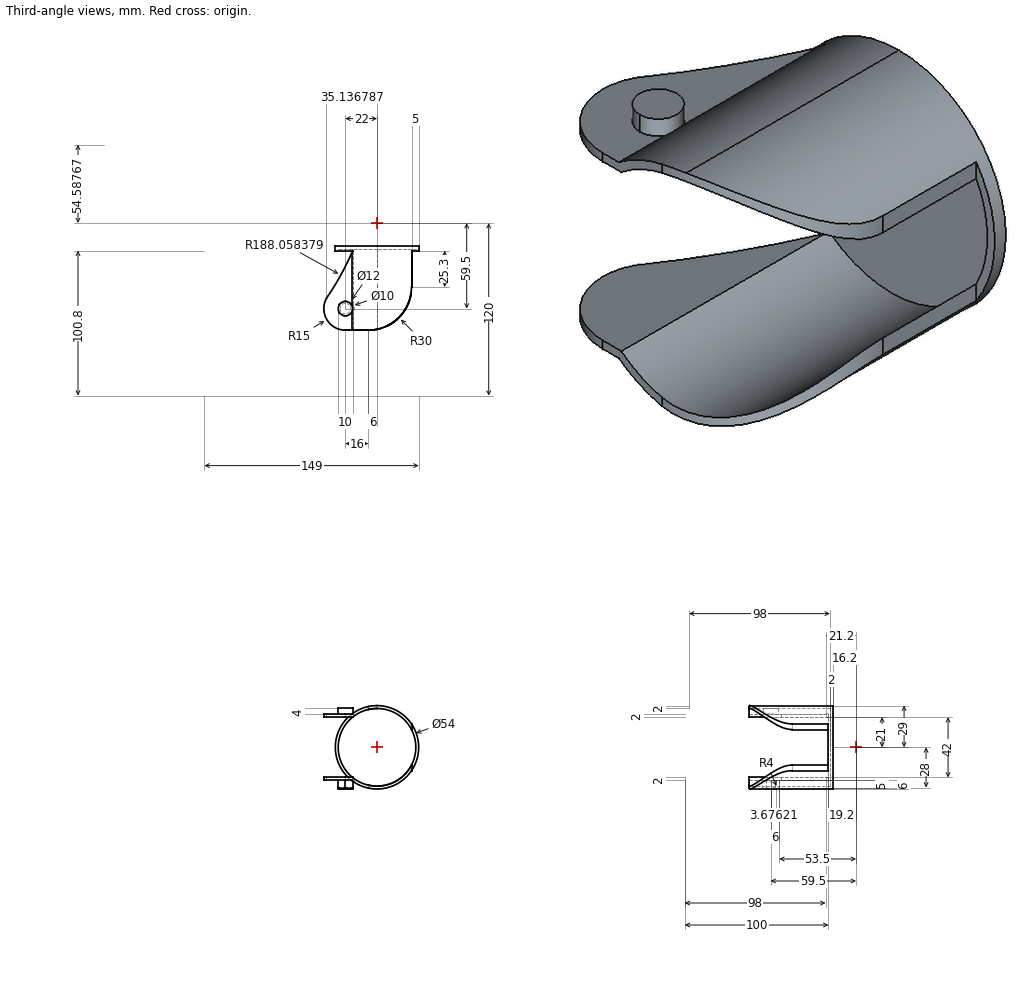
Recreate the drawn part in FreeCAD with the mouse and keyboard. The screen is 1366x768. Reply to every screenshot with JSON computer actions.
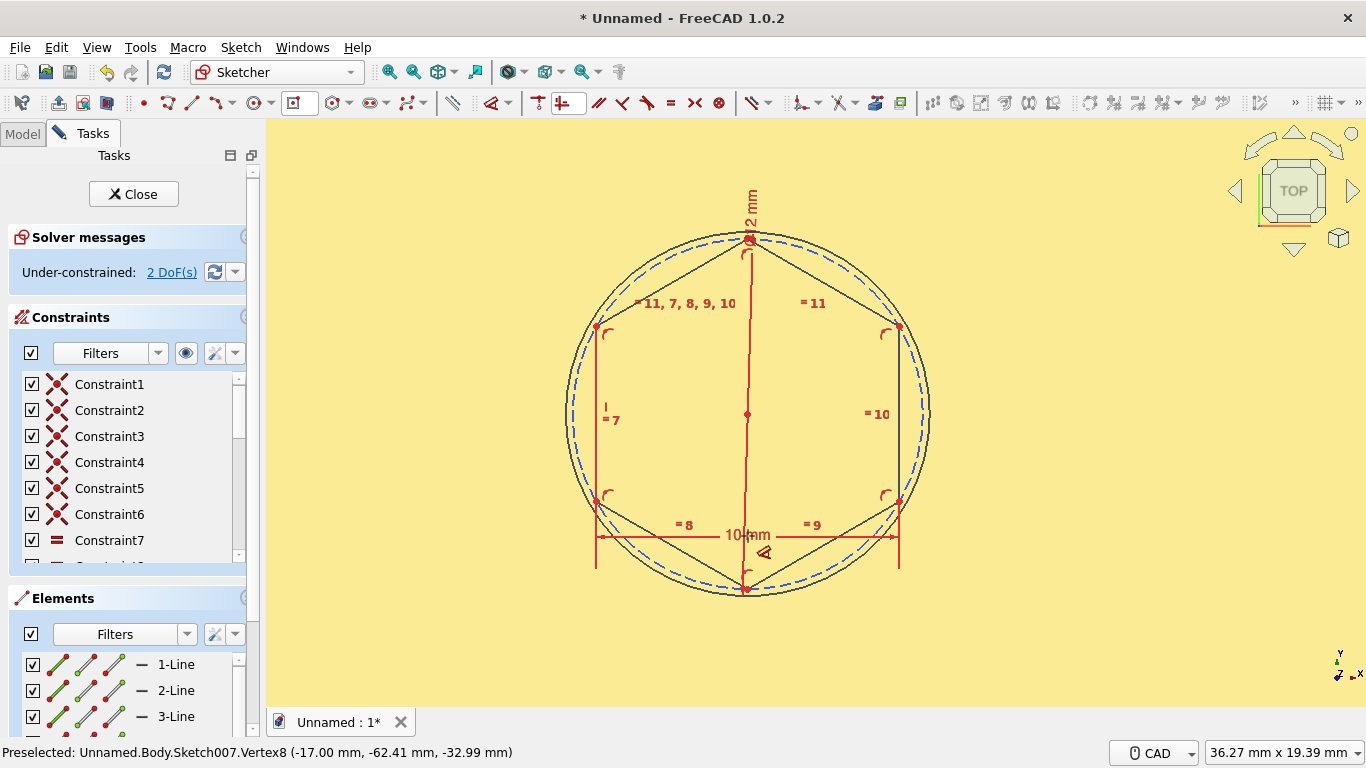
{"action": "left_click", "coordinate": [748, 414]}
{"action": "left_click", "coordinate": [974, 448]}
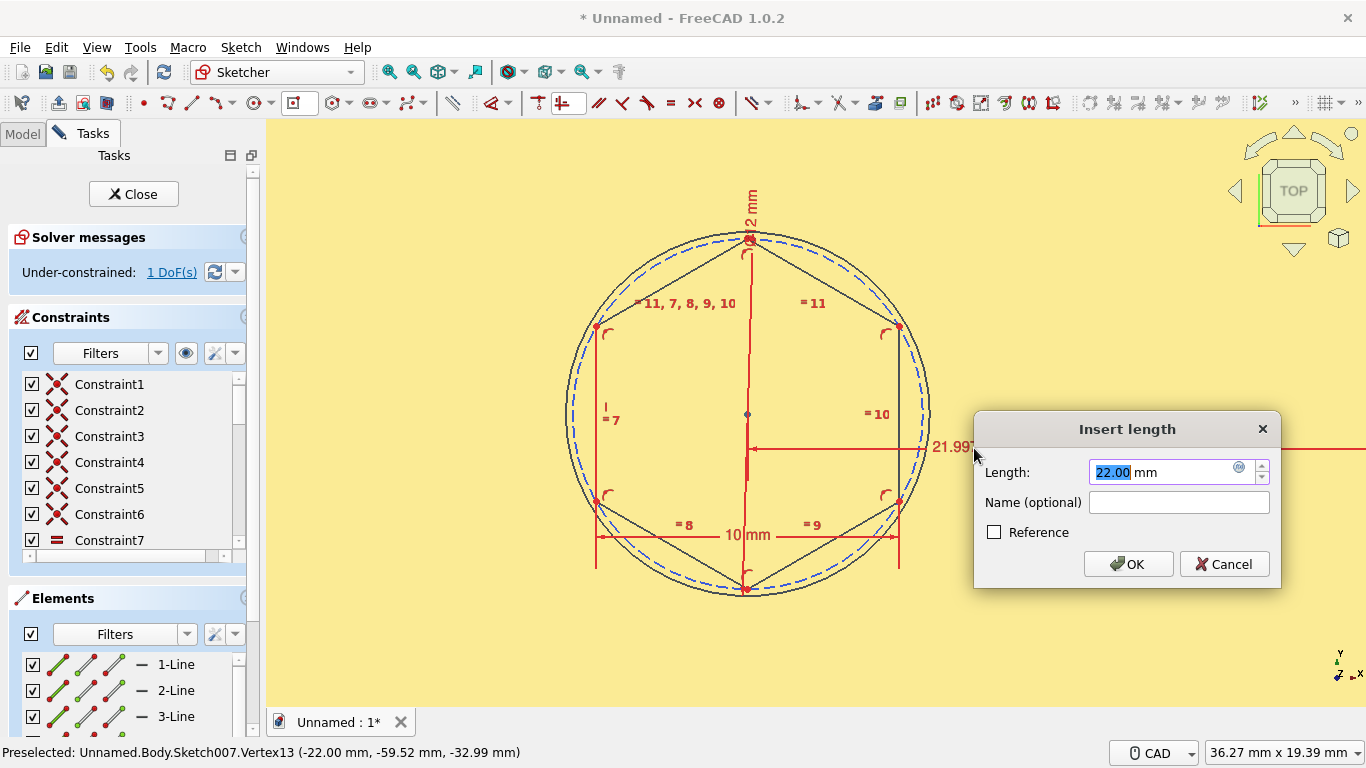
{"action": "type", "text": "22"}
{"action": "key", "text": "Return"}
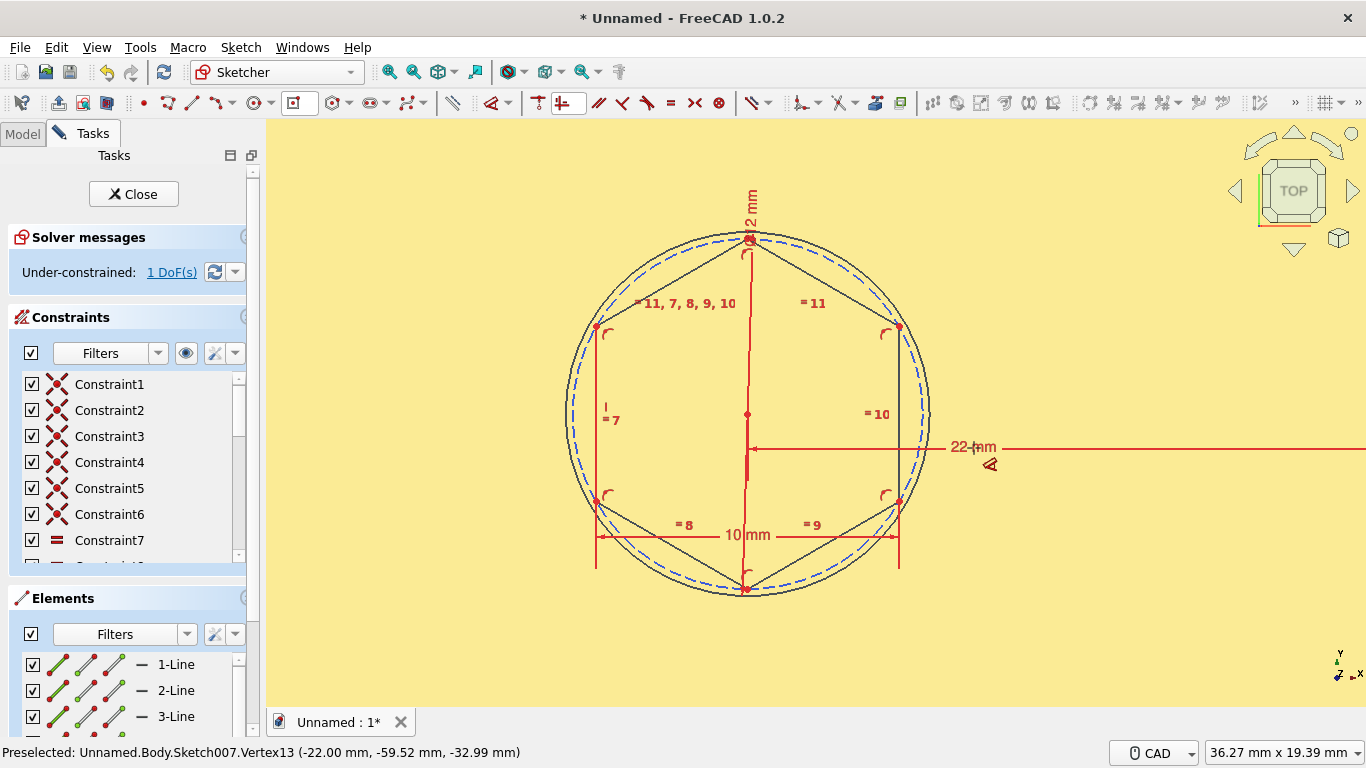
{"action": "left_click", "coordinate": [748, 414]}
{"action": "left_click", "coordinate": [714, 281]}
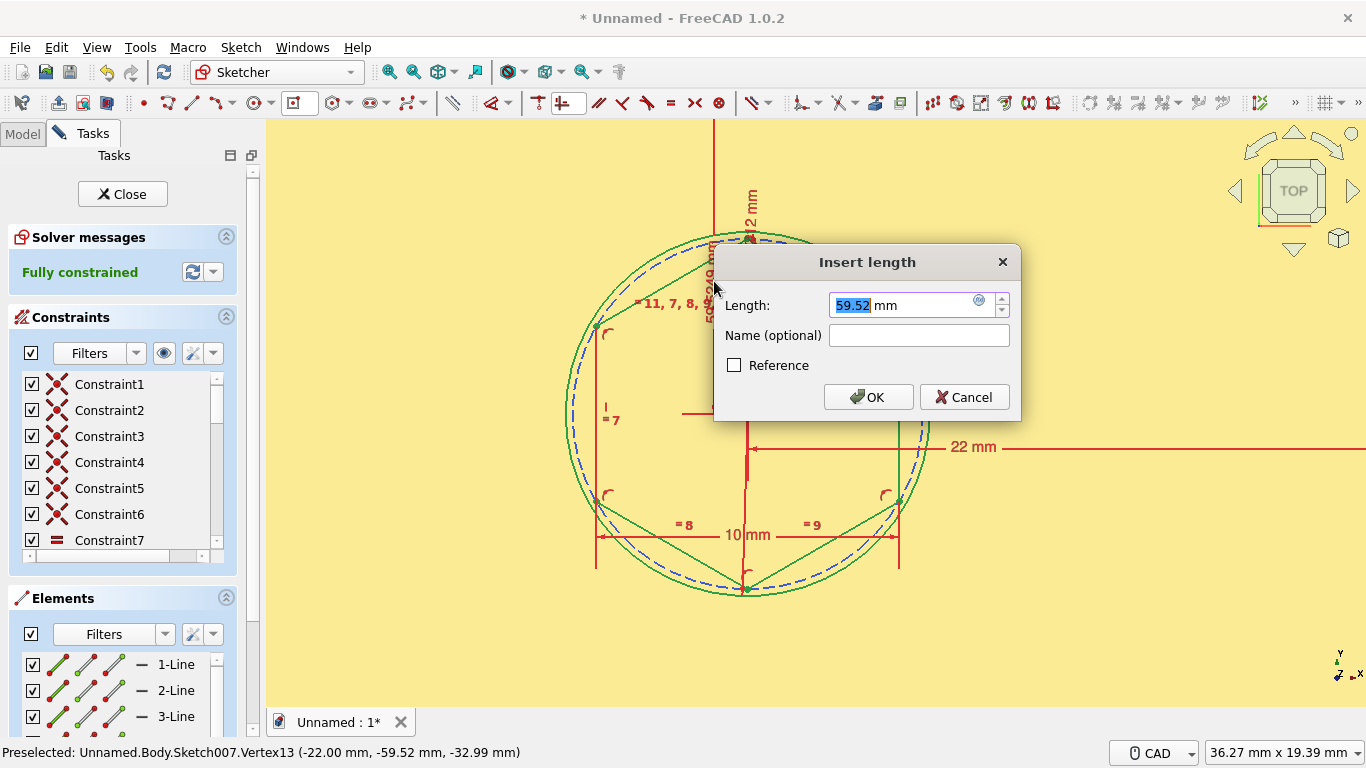
{"action": "type", "text": "59.5"}
{"action": "key", "text": "Return"}
{"action": "key", "text": "Escape"}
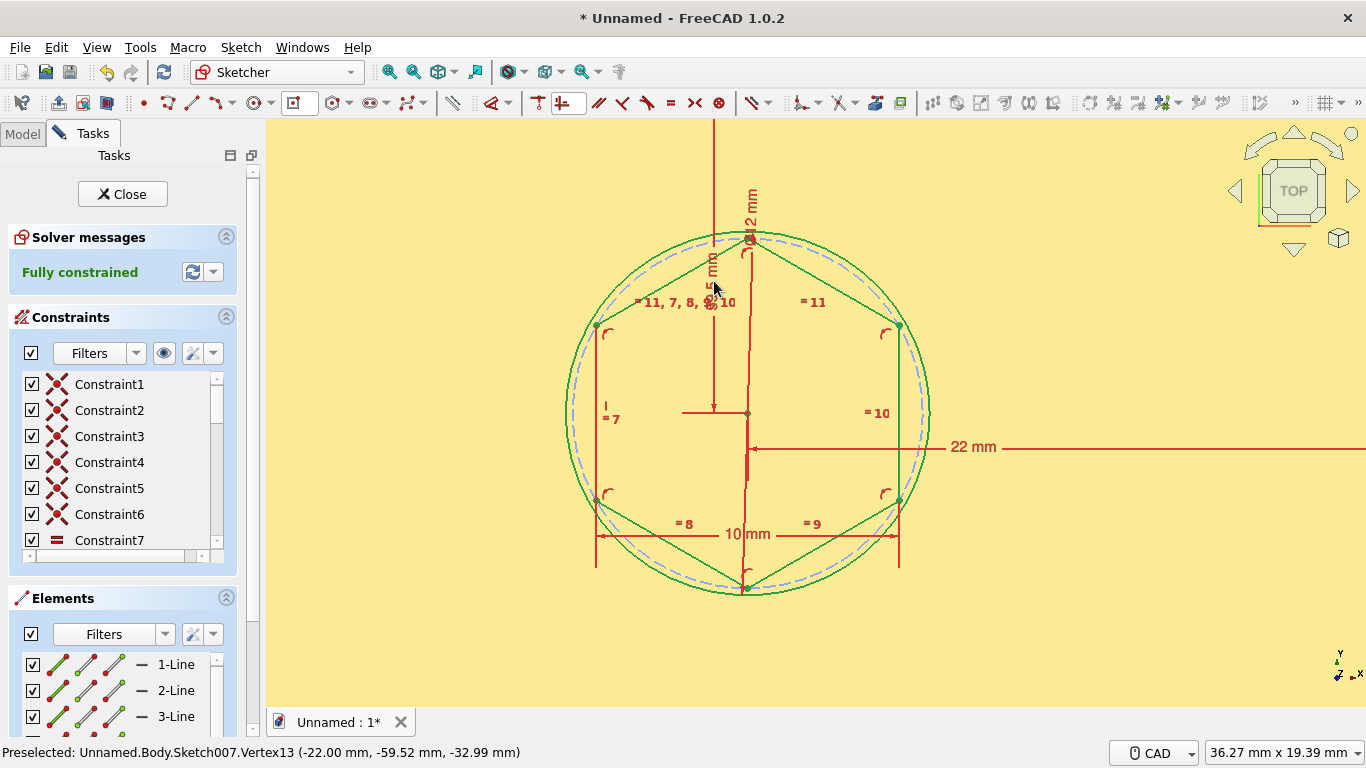
{"action": "left_click", "coordinate": [123, 194]}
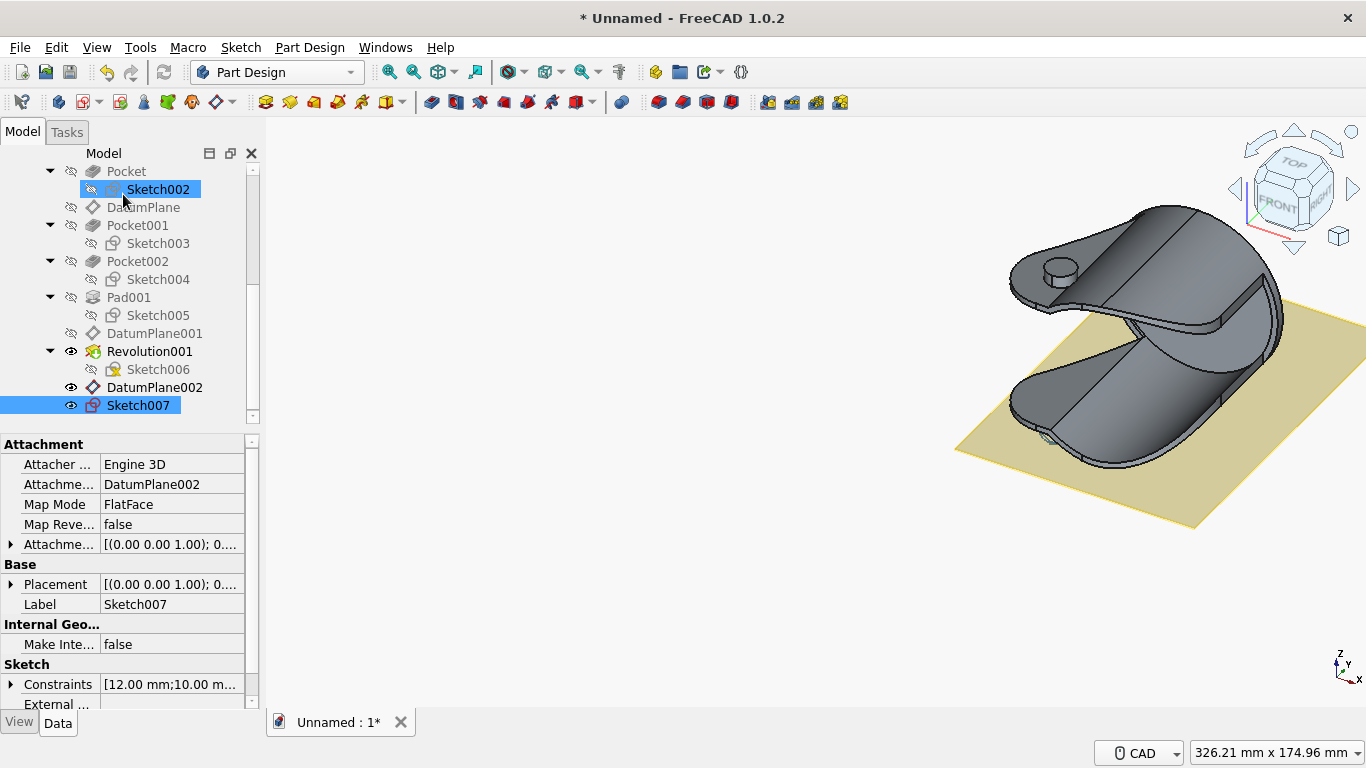
{"action": "left_click", "coordinate": [432, 102]}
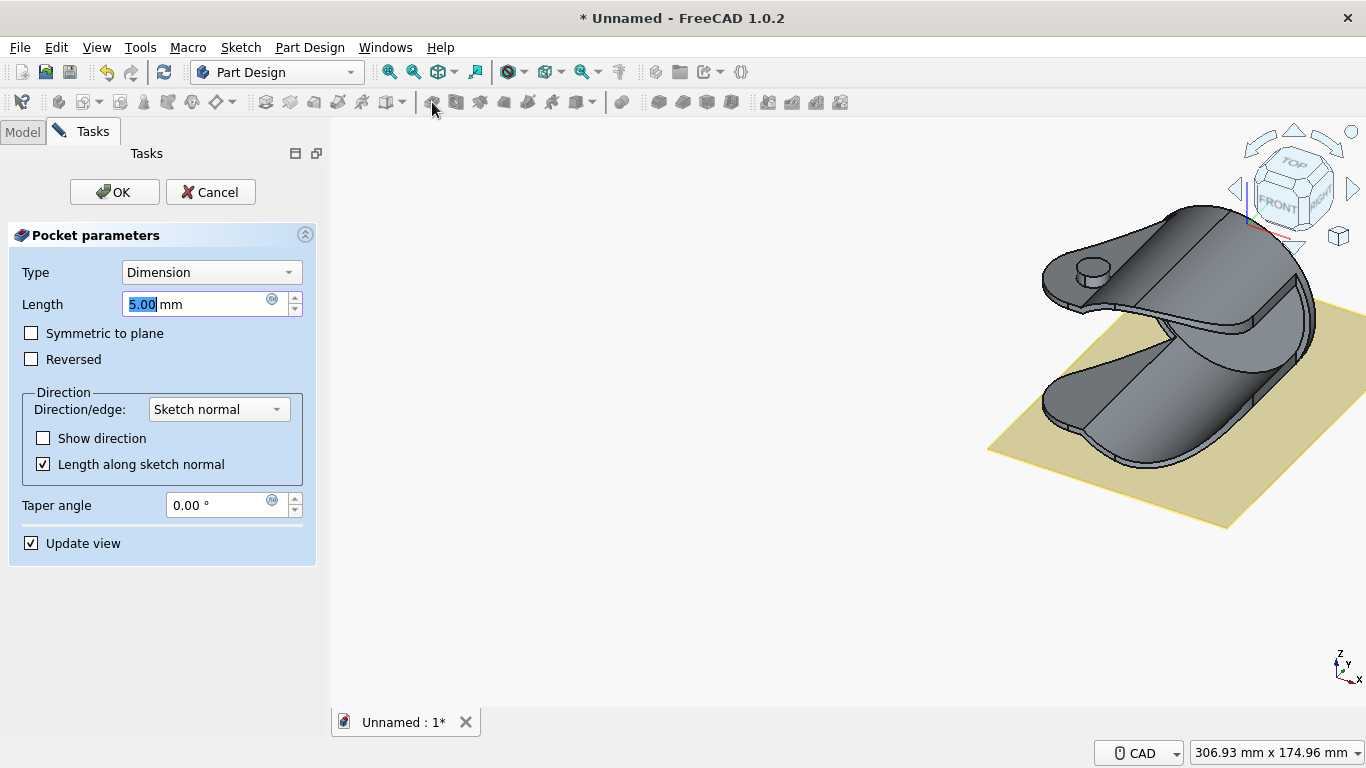
{"action": "type", "text": "10"}
{"action": "key", "text": "Tab"}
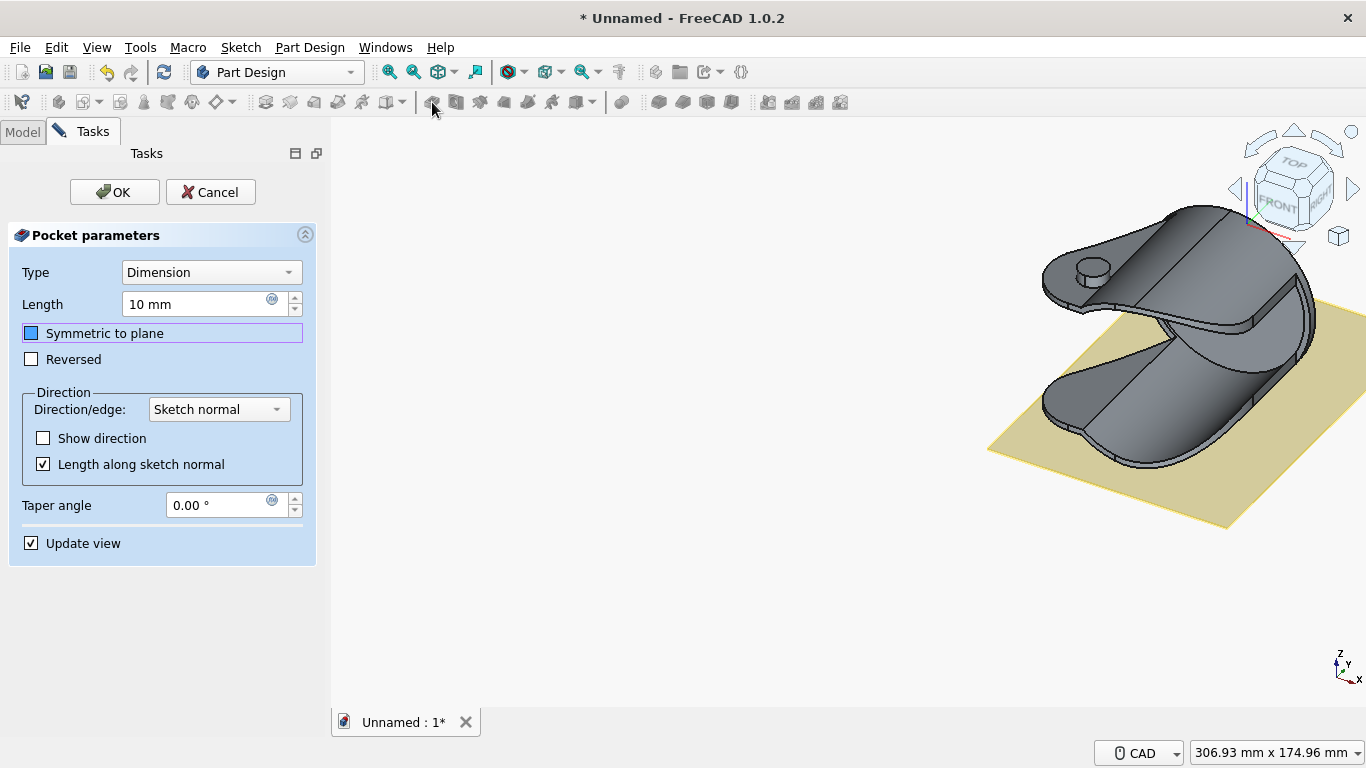
{"action": "left_click", "coordinate": [30, 359]}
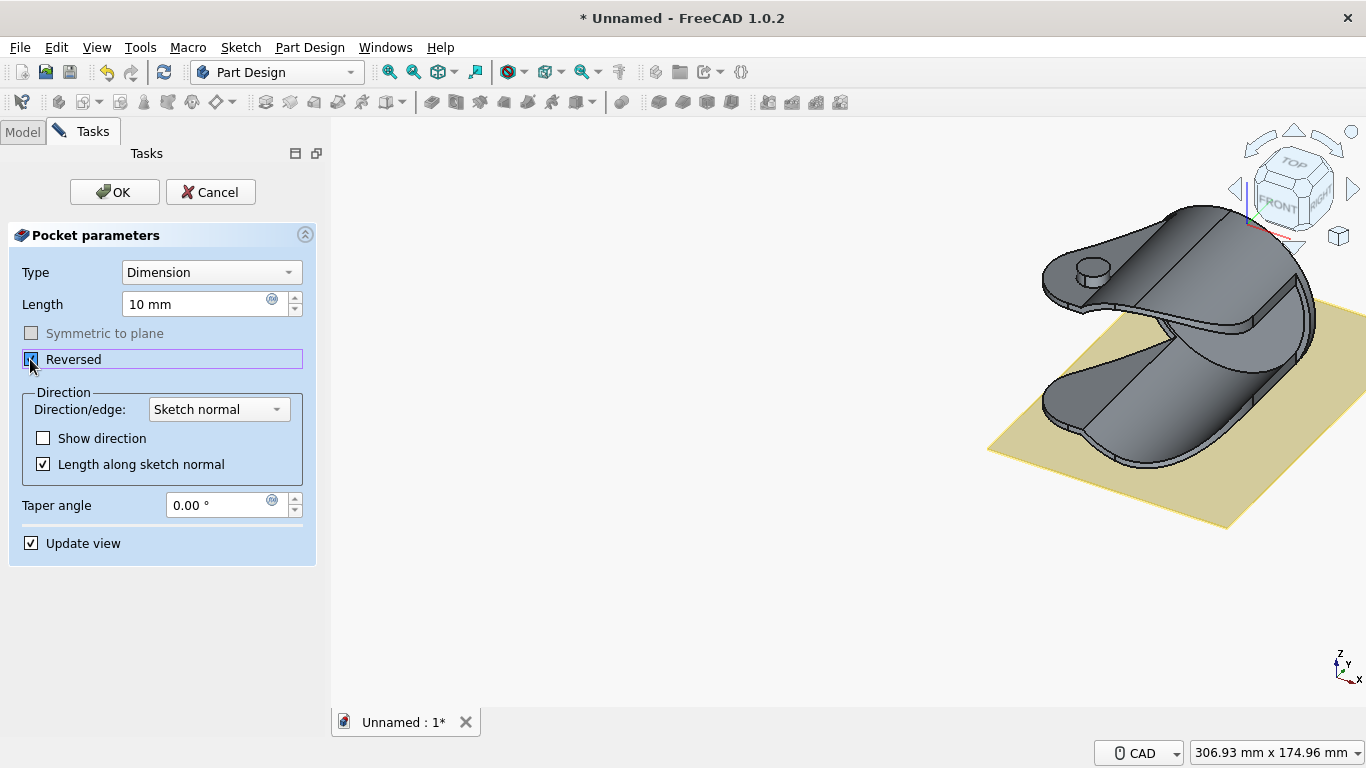
{"action": "left_click", "coordinate": [115, 192]}